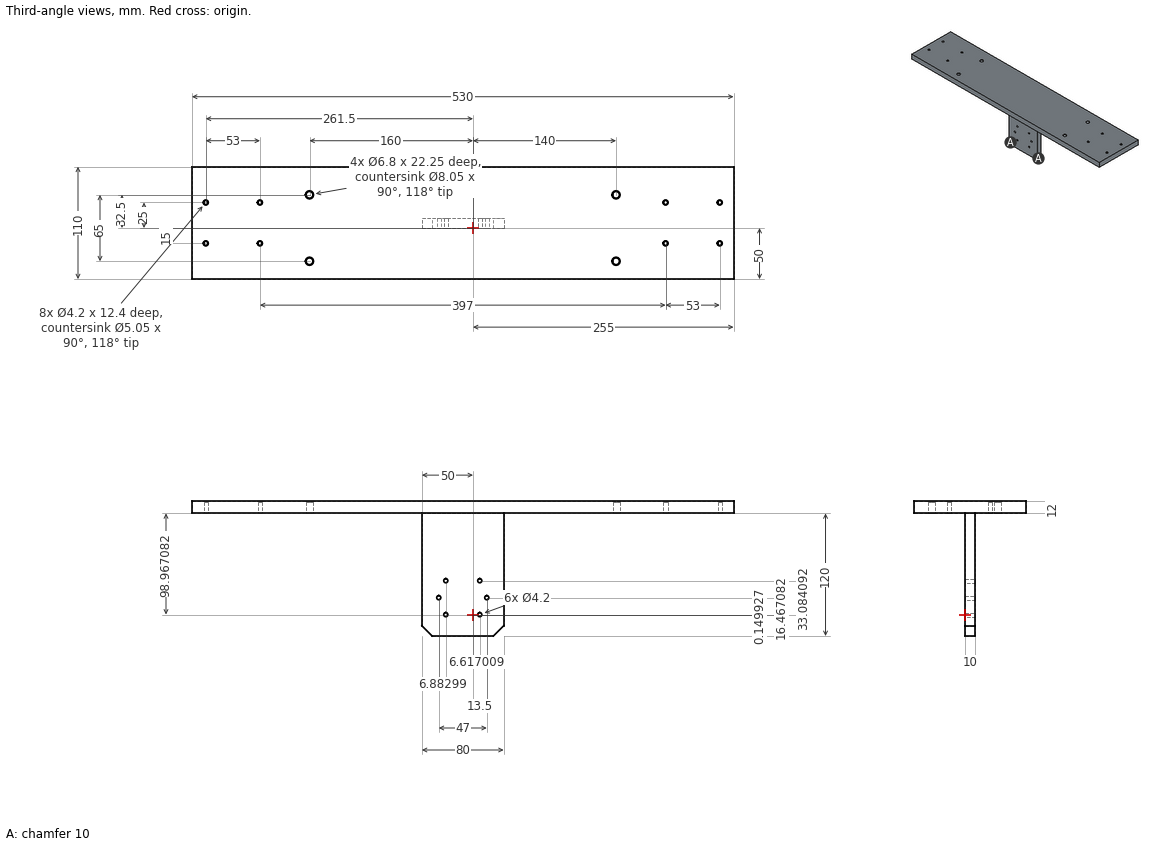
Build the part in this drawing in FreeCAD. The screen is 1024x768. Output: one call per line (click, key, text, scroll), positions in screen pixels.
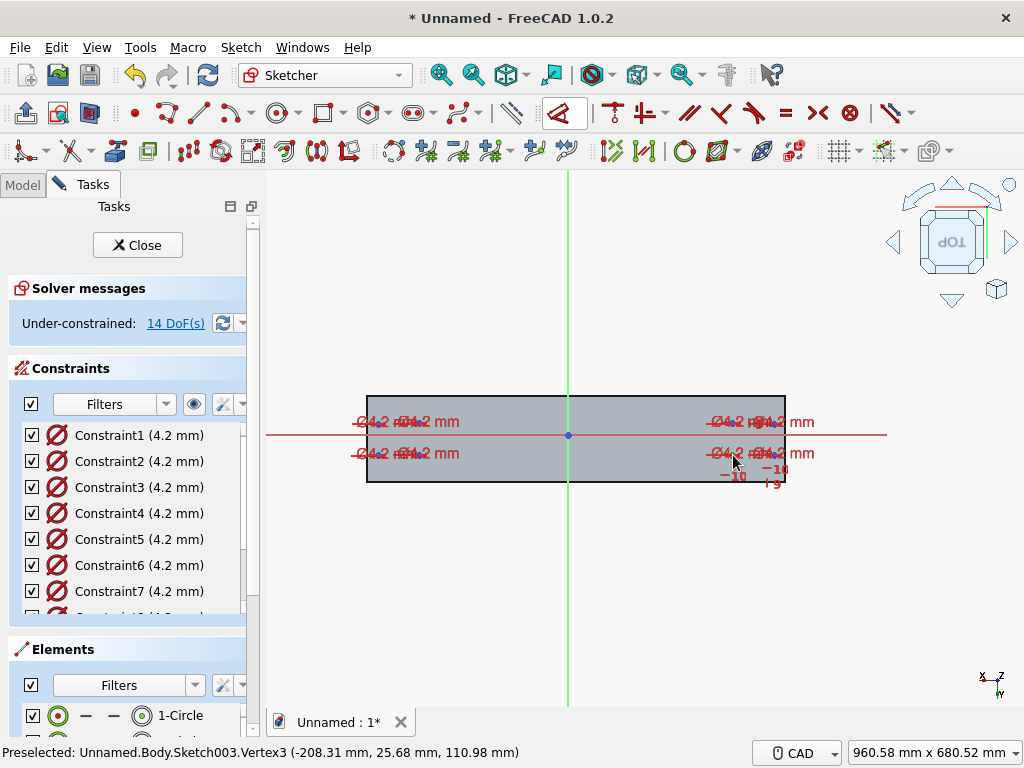
click(733, 424)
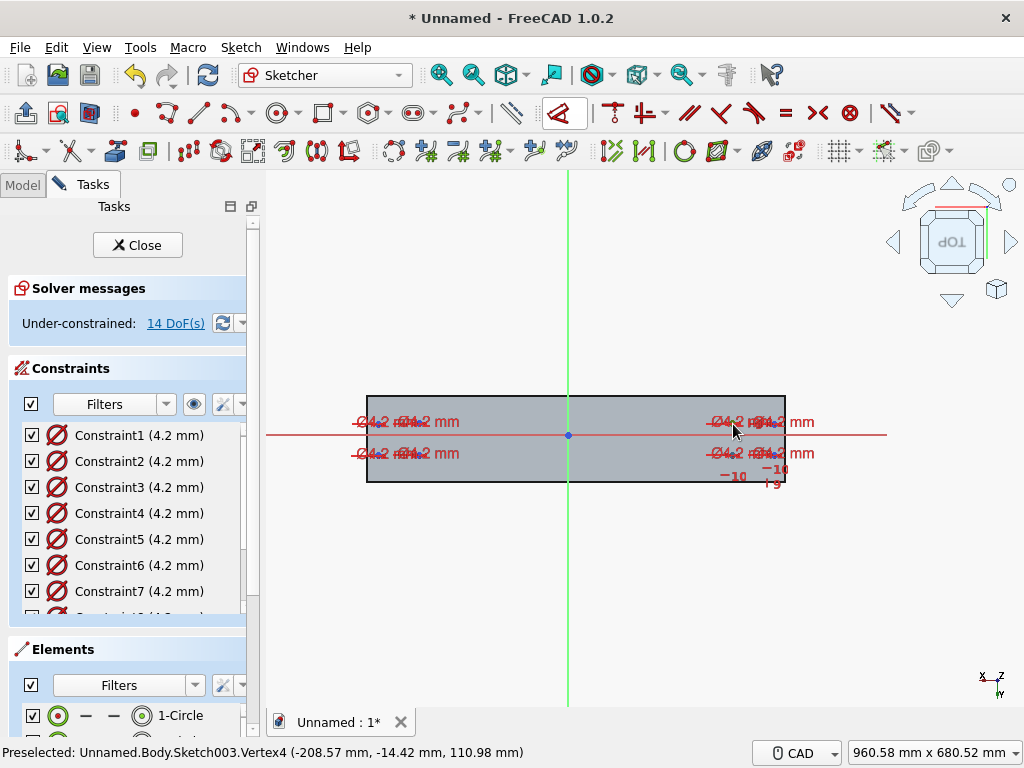
key(v)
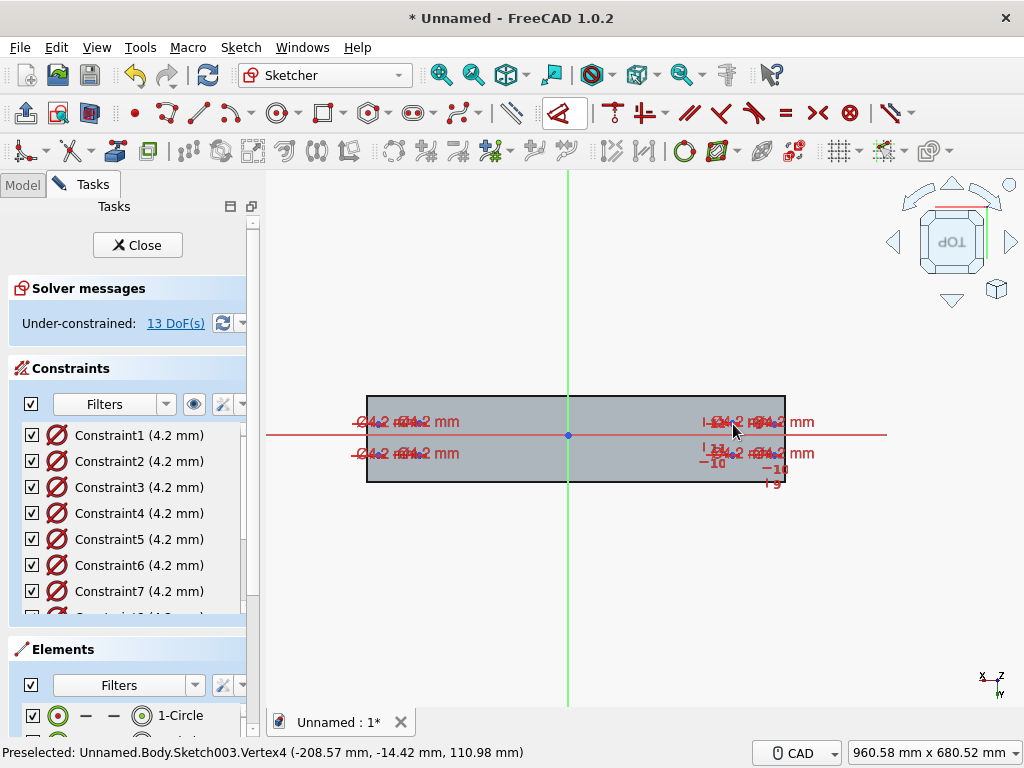
click(775, 424)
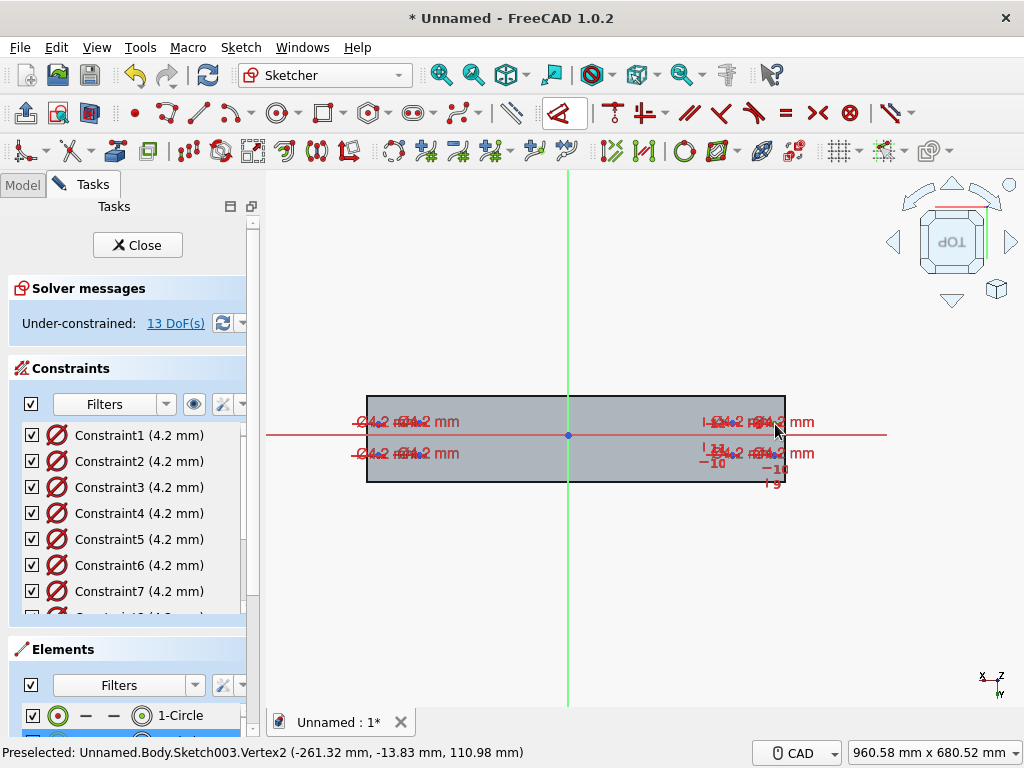
click(733, 424)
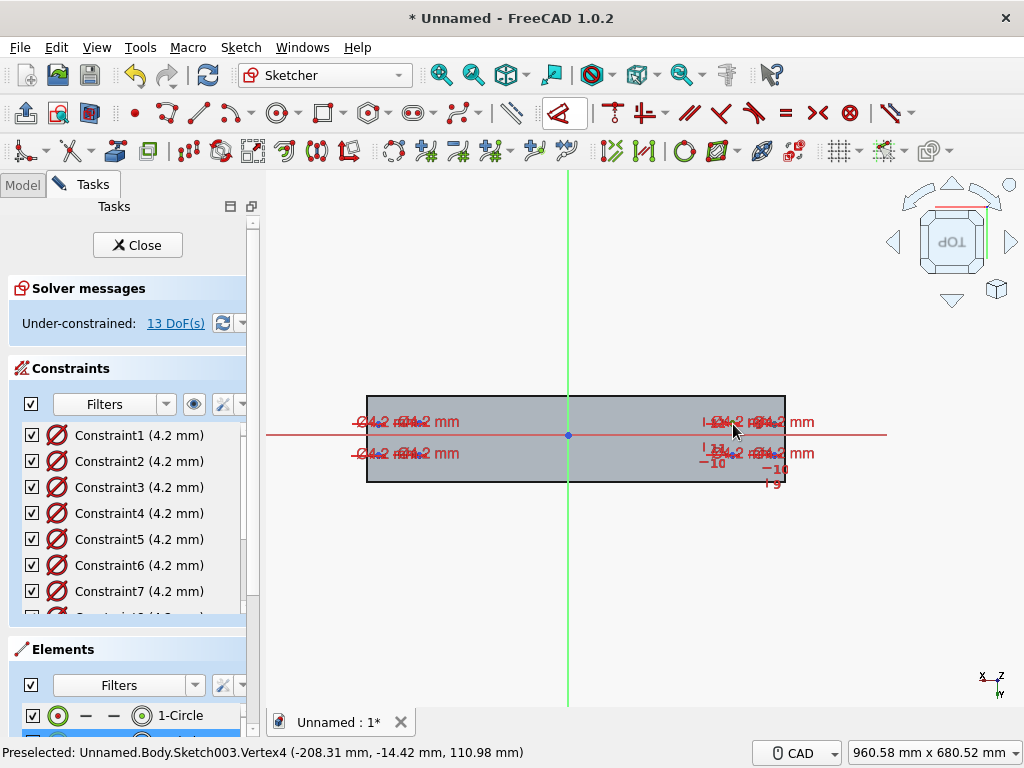
key(h)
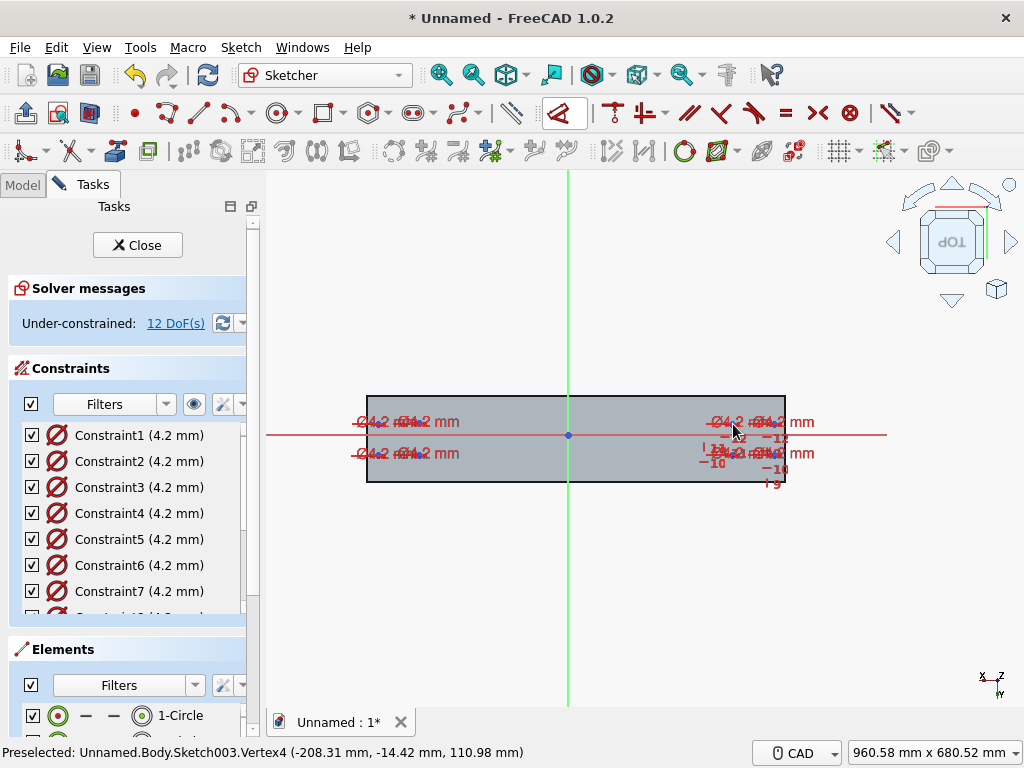
click(733, 424)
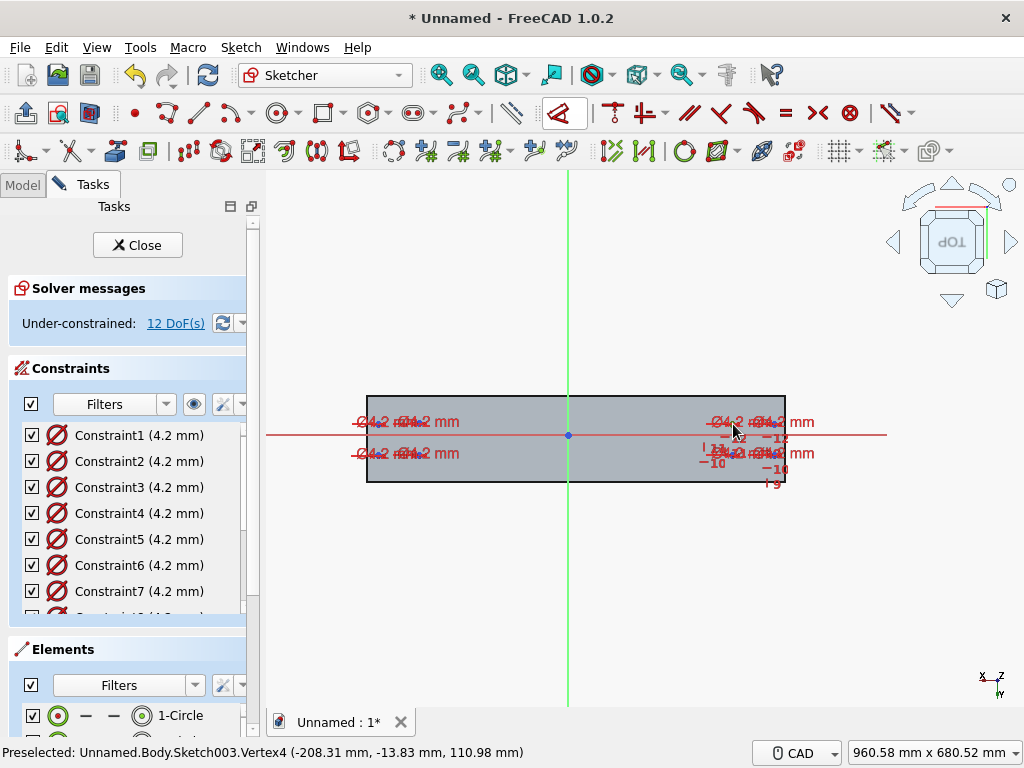
click(419, 424)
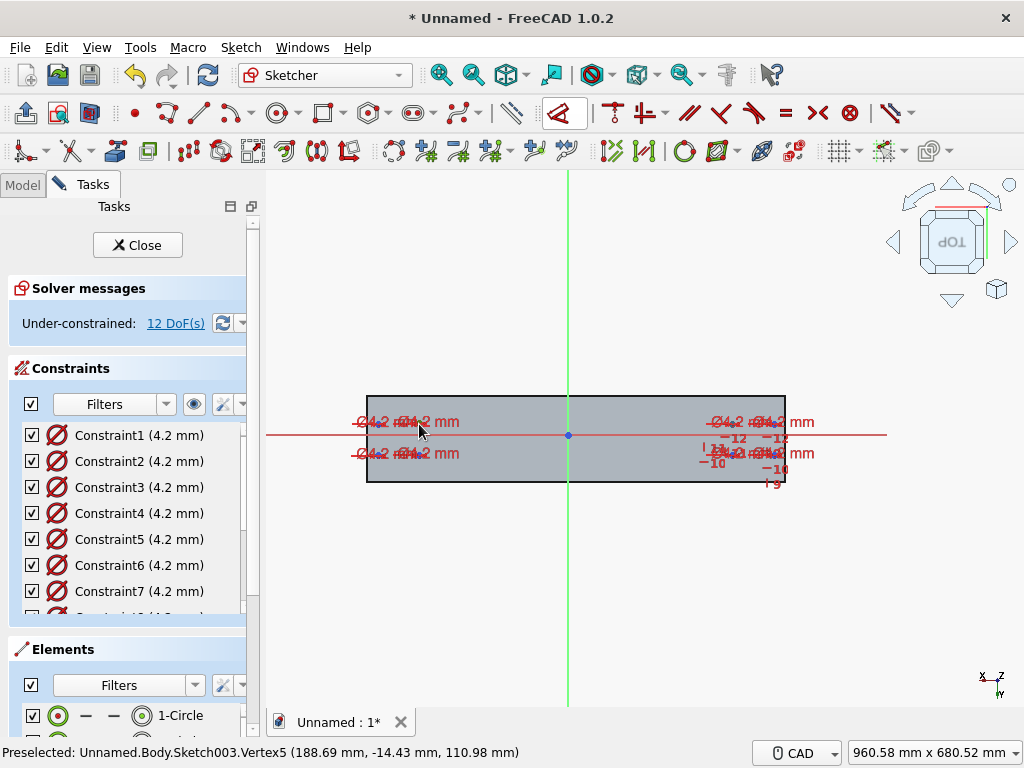
key(h)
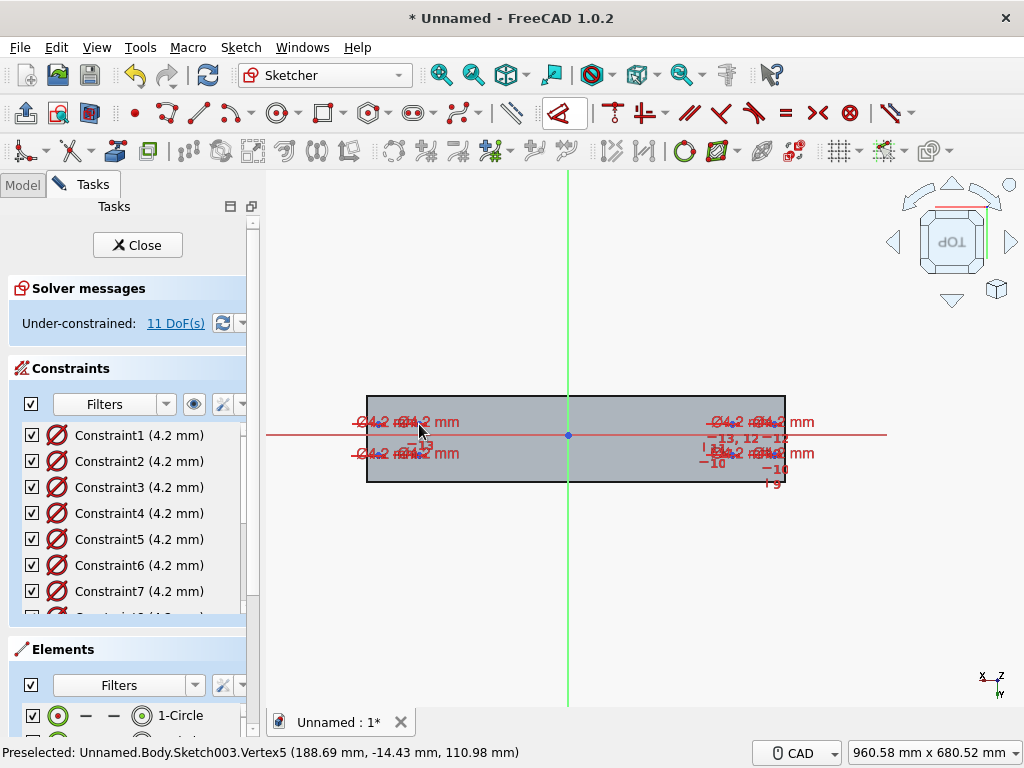
click(419, 424)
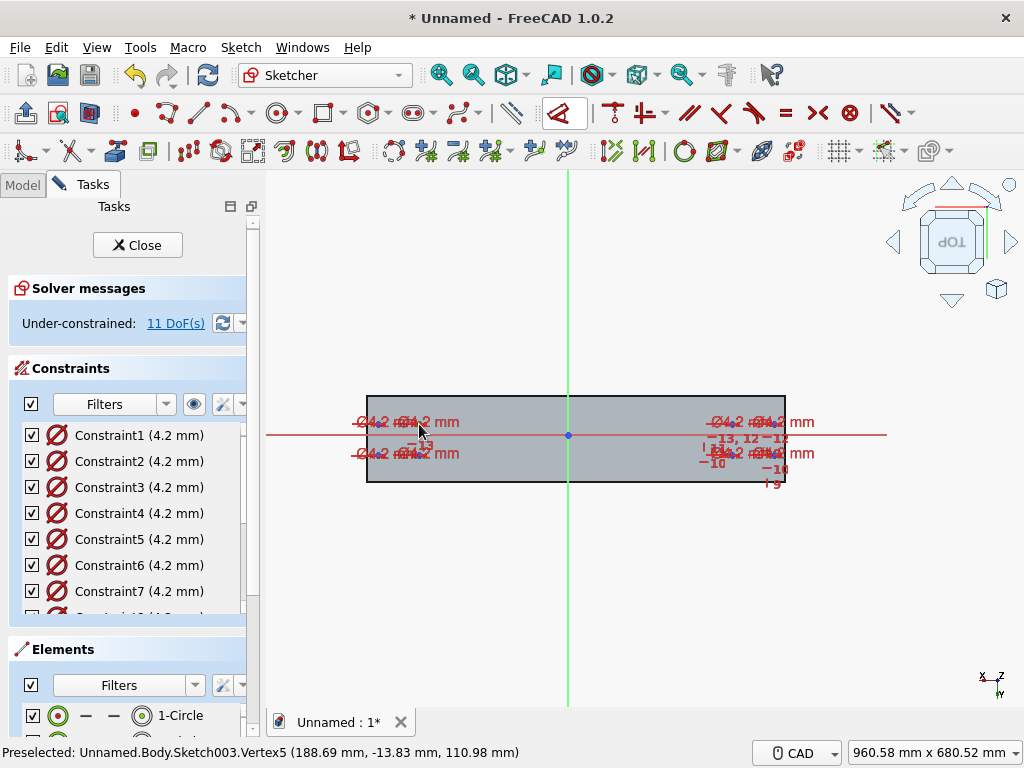
click(419, 455)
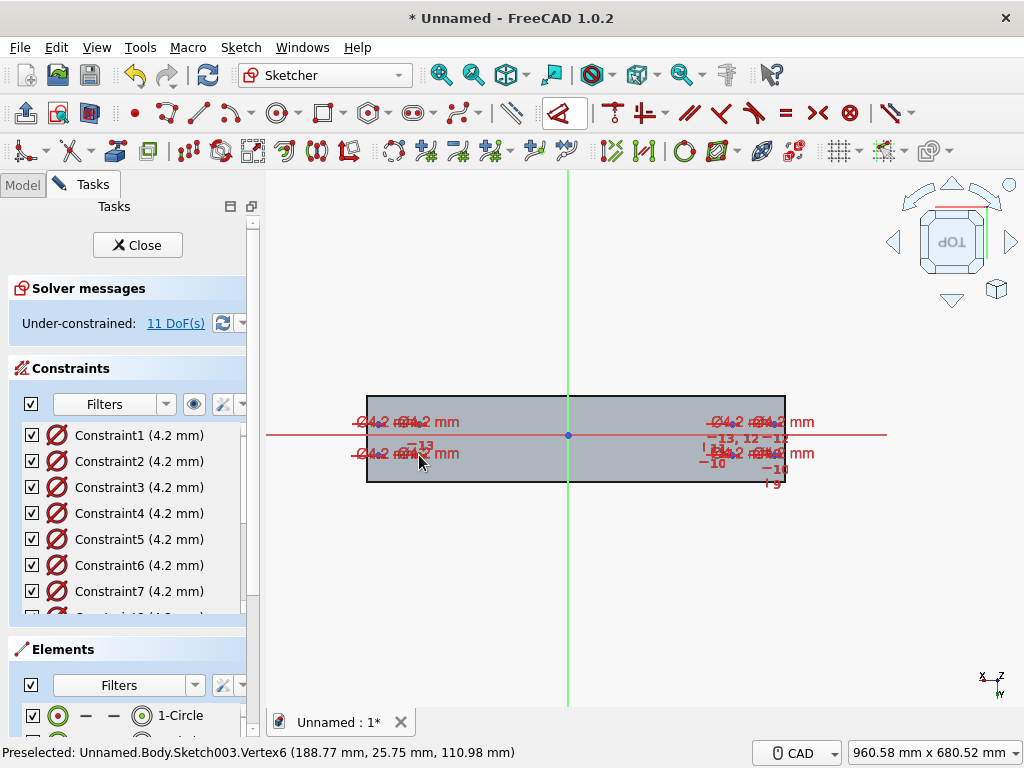
key(v)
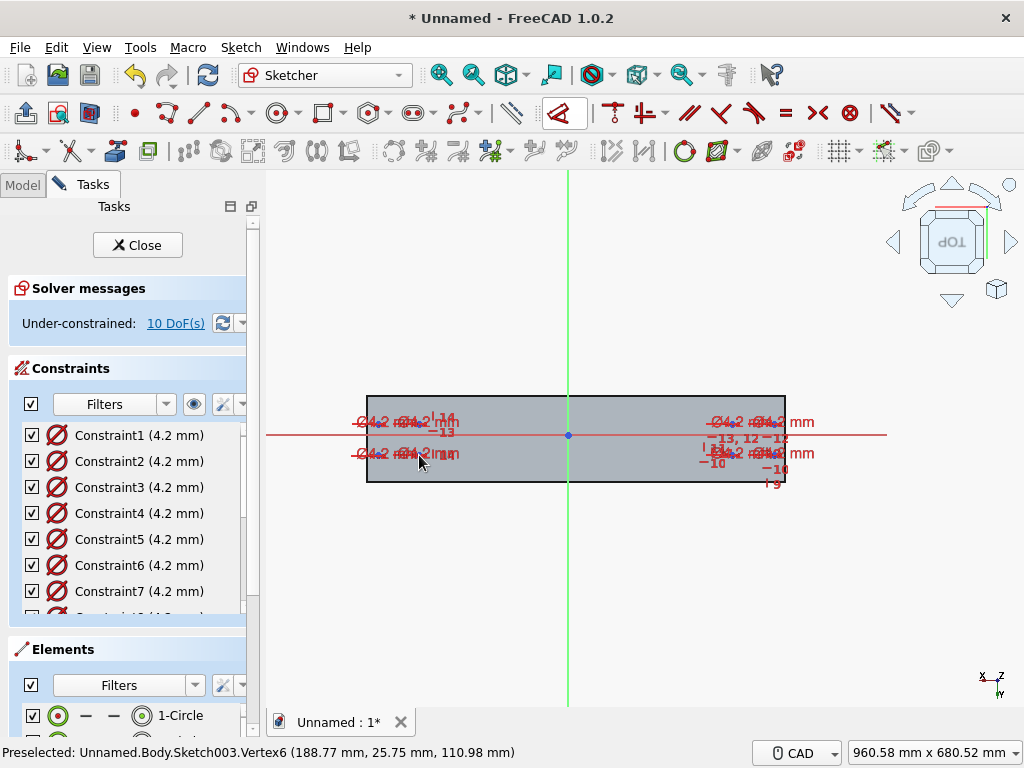
click(733, 455)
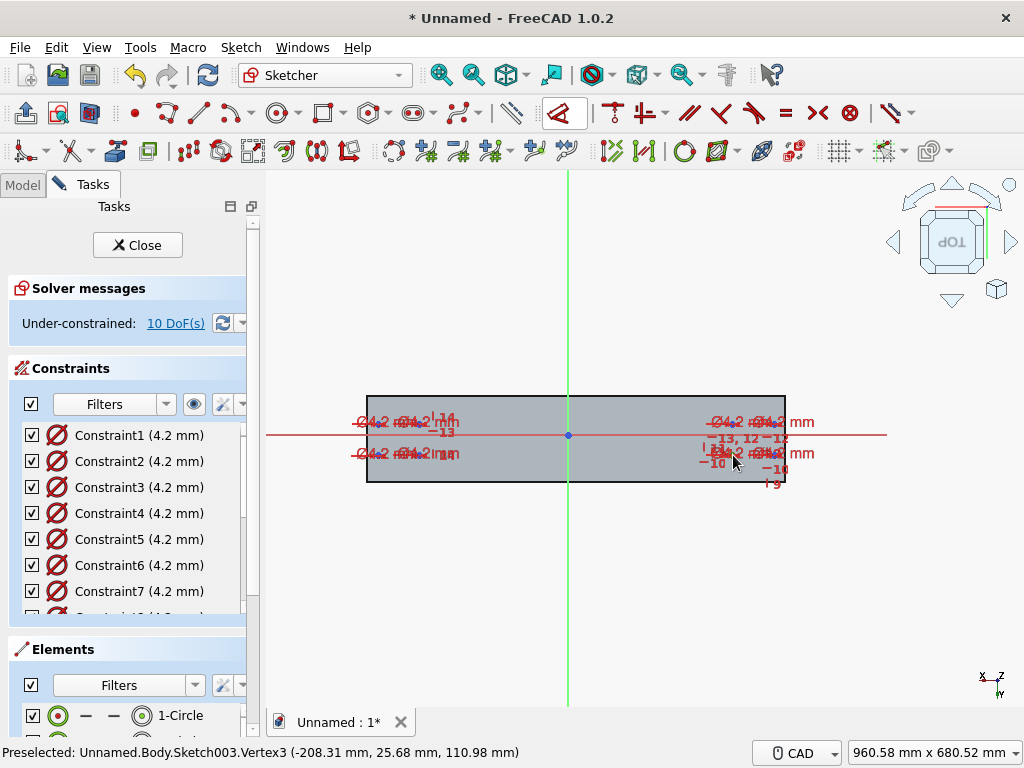
click(419, 455)